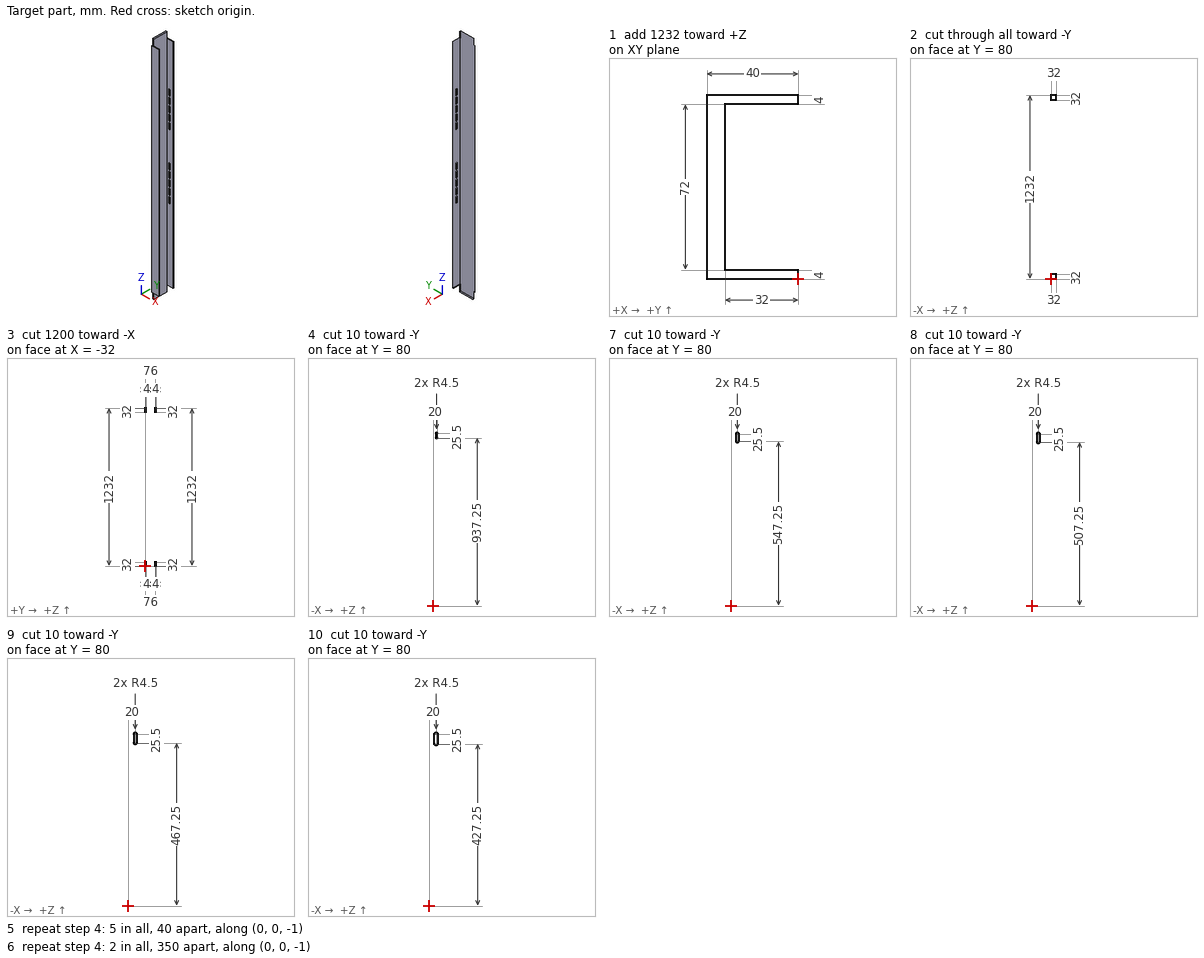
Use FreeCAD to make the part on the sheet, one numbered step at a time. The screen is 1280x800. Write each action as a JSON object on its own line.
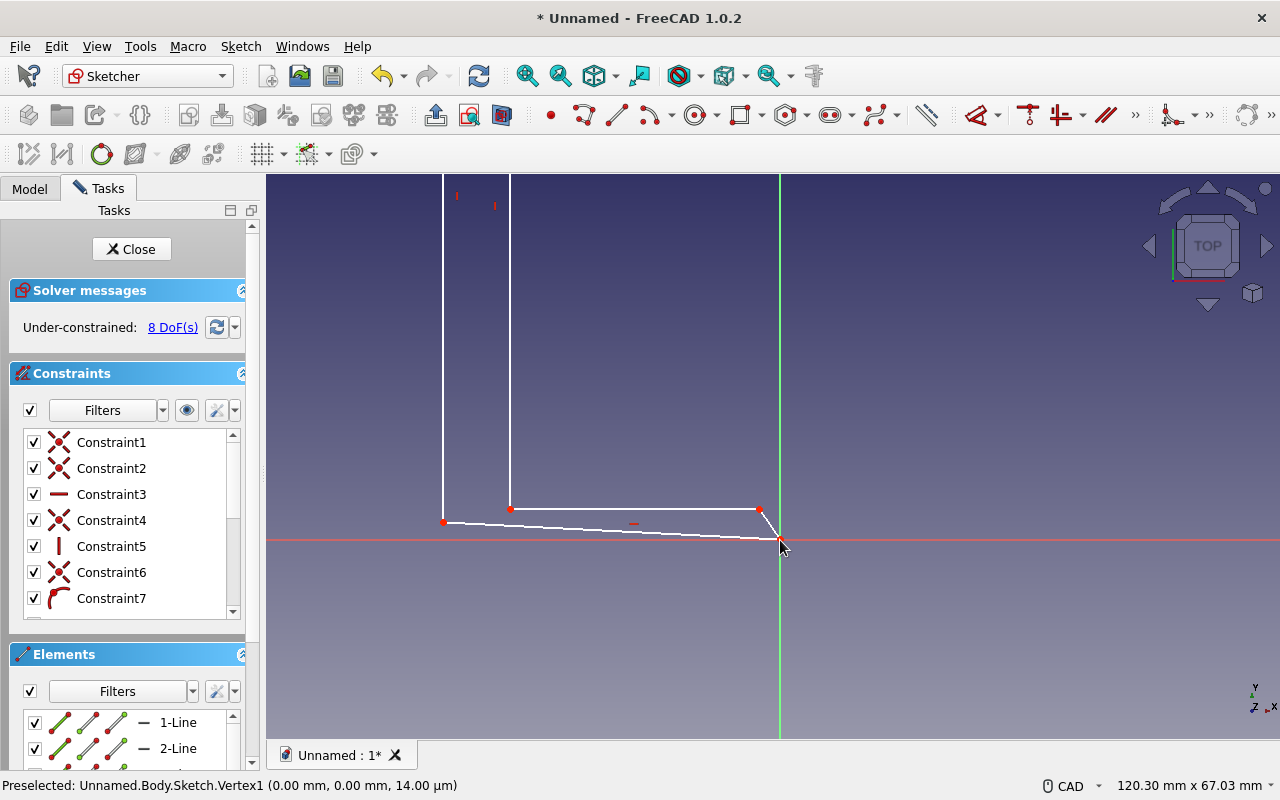
{"action": "scroll", "coordinate": [766, 518], "scroll_direction": "up", "scroll_amount": 2}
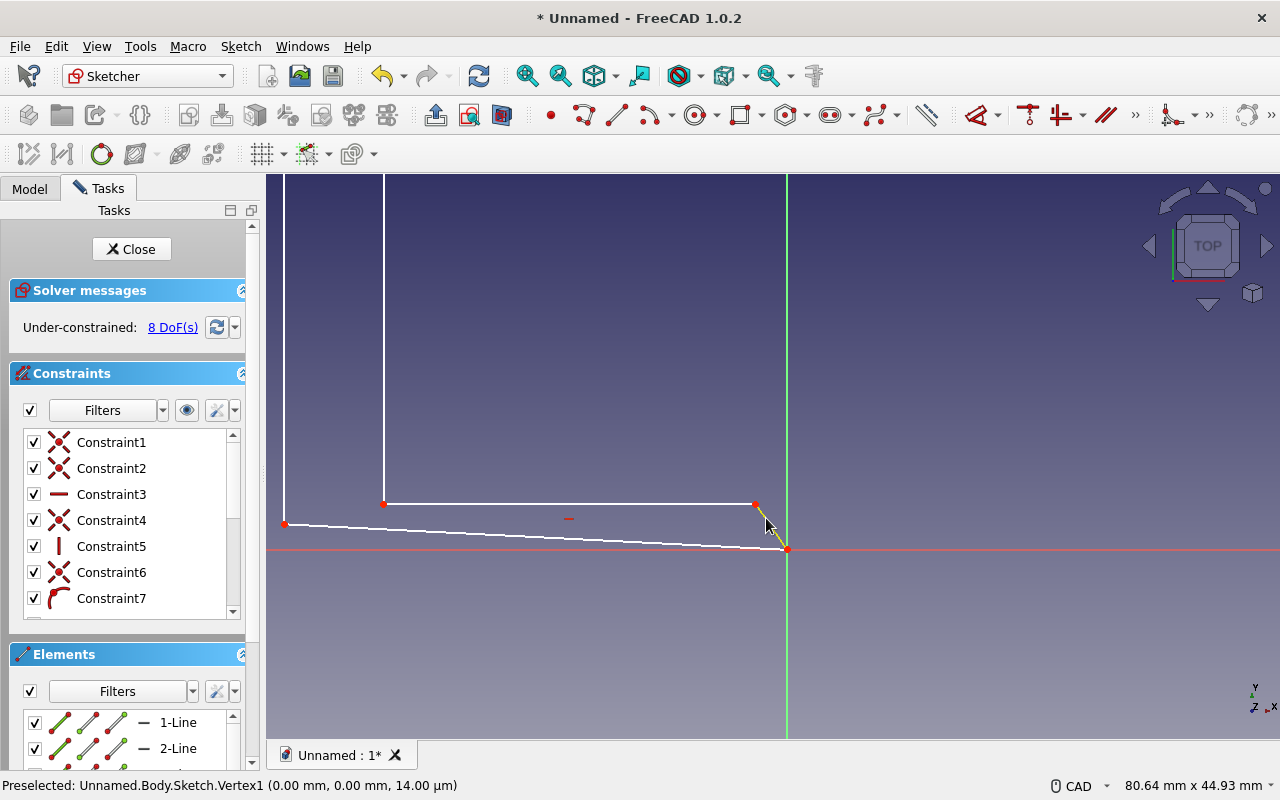
{"action": "left_click", "coordinate": [765, 518]}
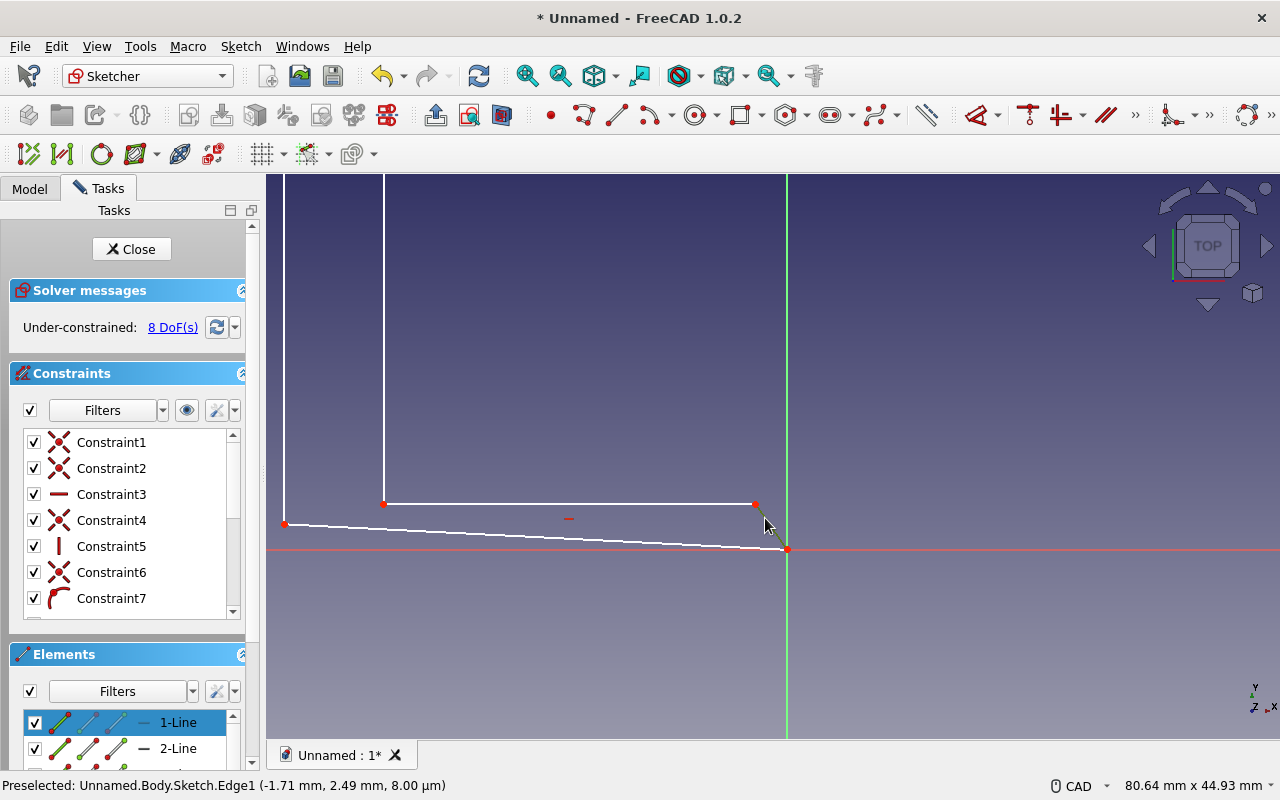
{"action": "key", "text": "v"}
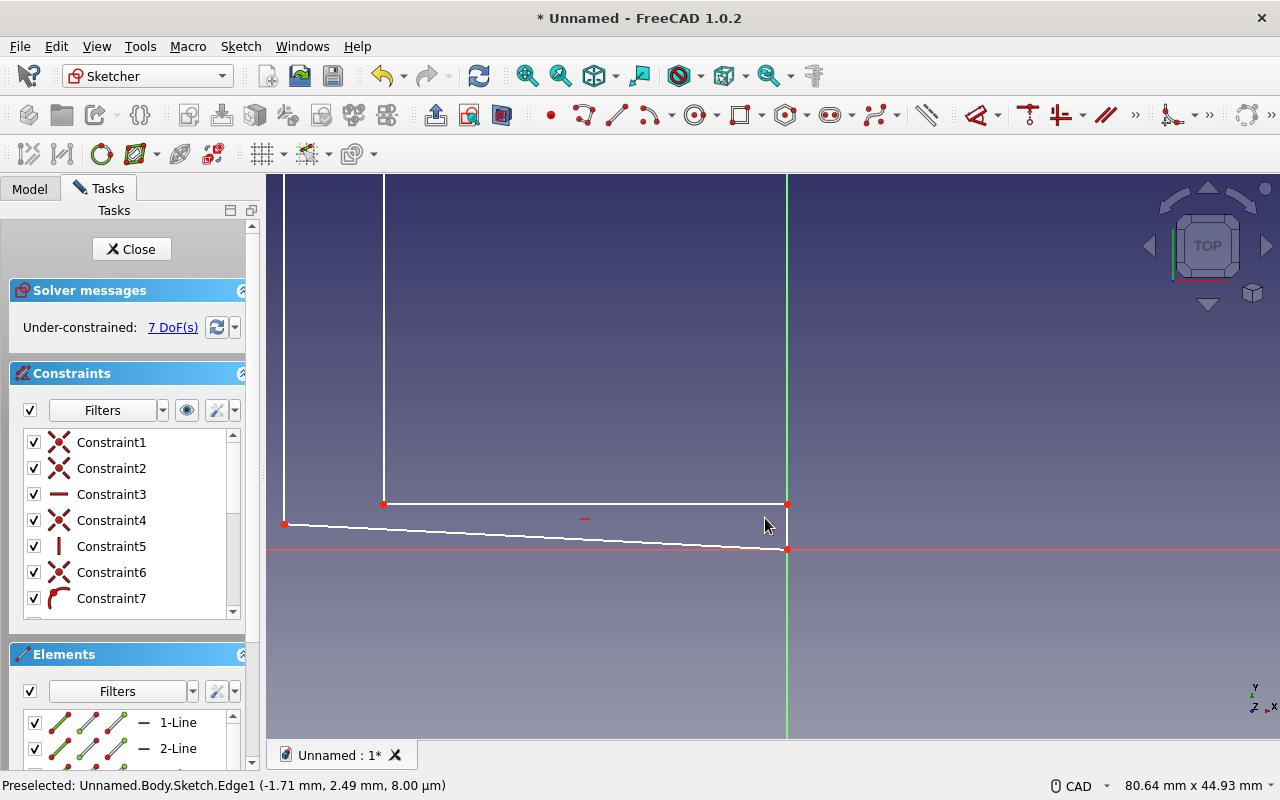
{"action": "scroll", "coordinate": [803, 695], "scroll_direction": "down", "scroll_amount": 5}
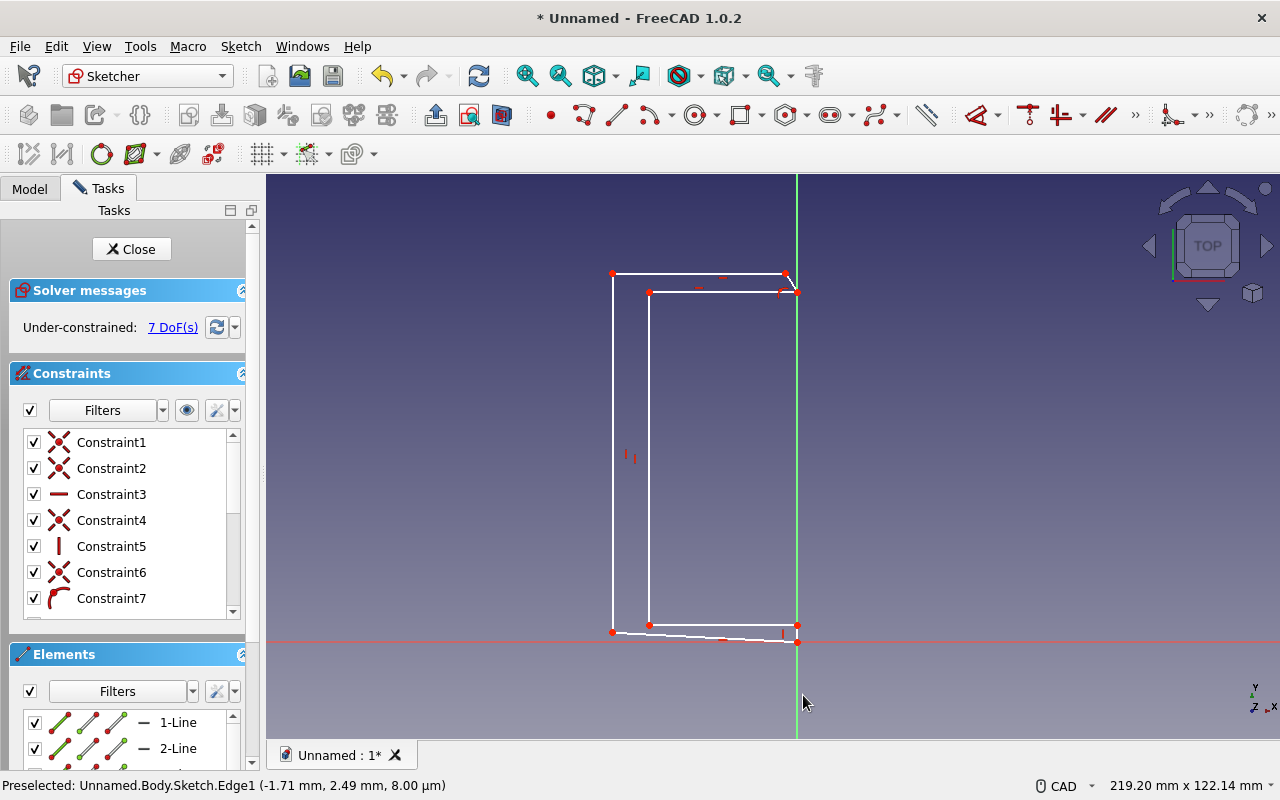
{"action": "scroll", "coordinate": [794, 287], "scroll_direction": "up", "scroll_amount": 7}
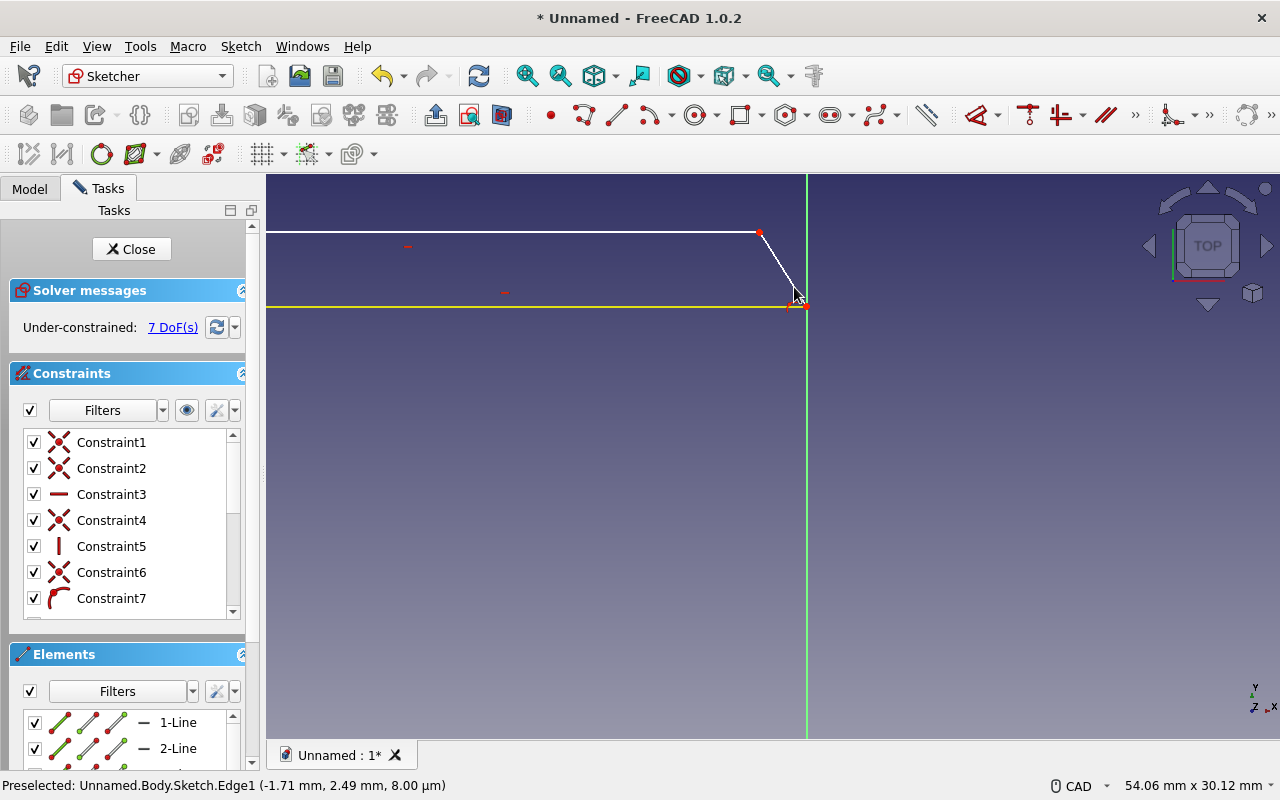
{"action": "left_click", "coordinate": [793, 284]}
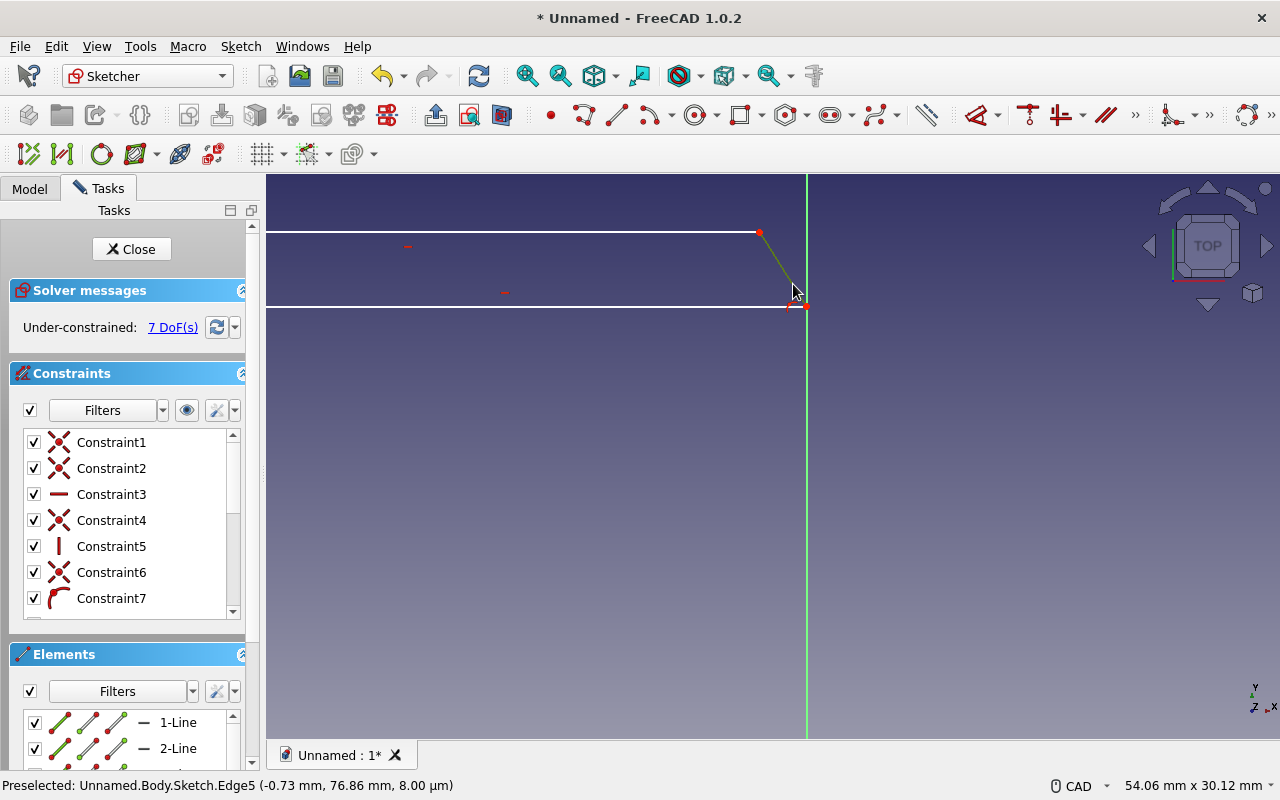
{"action": "left_click", "coordinate": [1082, 116]}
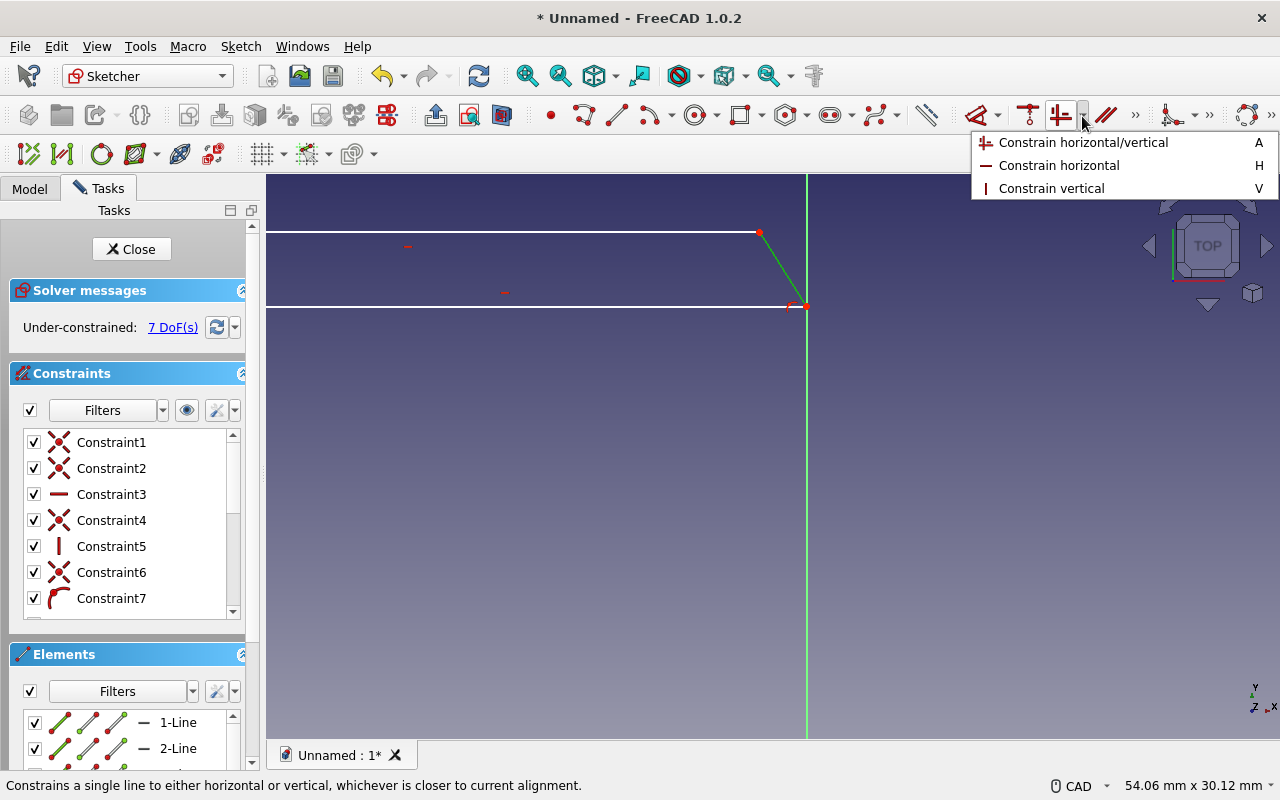
{"action": "left_click", "coordinate": [1125, 188]}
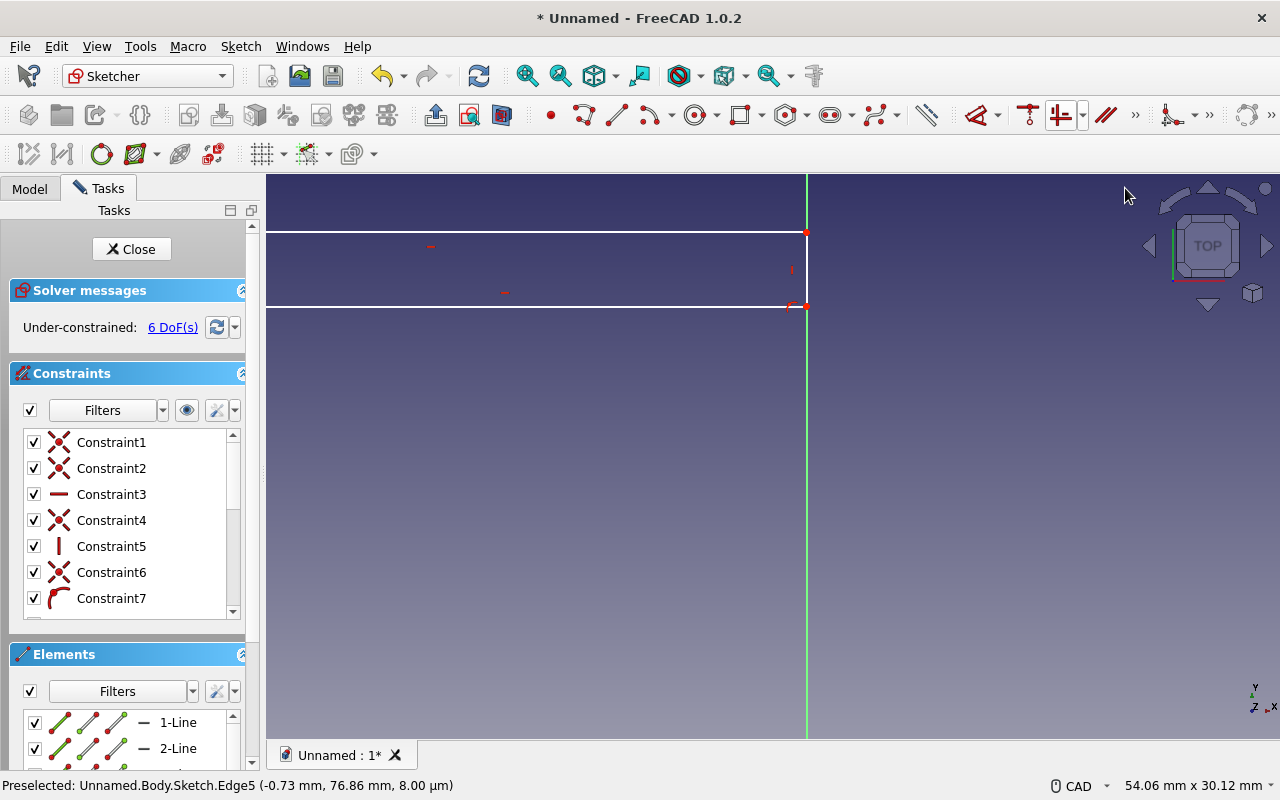
{"action": "scroll", "coordinate": [794, 286], "scroll_direction": "down", "scroll_amount": 7}